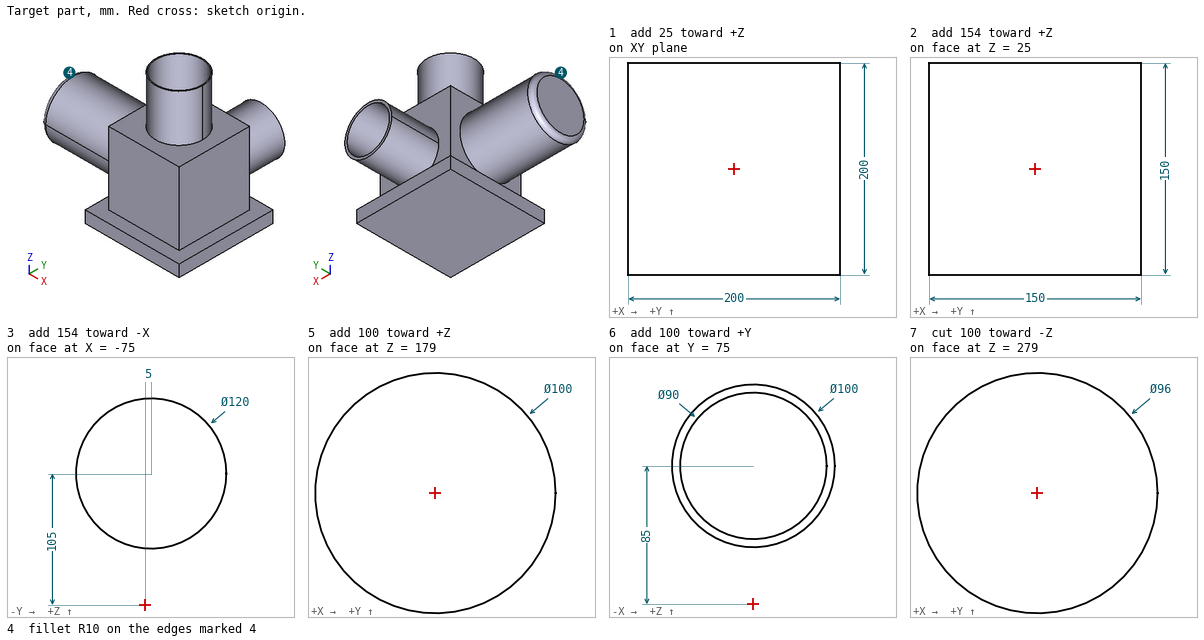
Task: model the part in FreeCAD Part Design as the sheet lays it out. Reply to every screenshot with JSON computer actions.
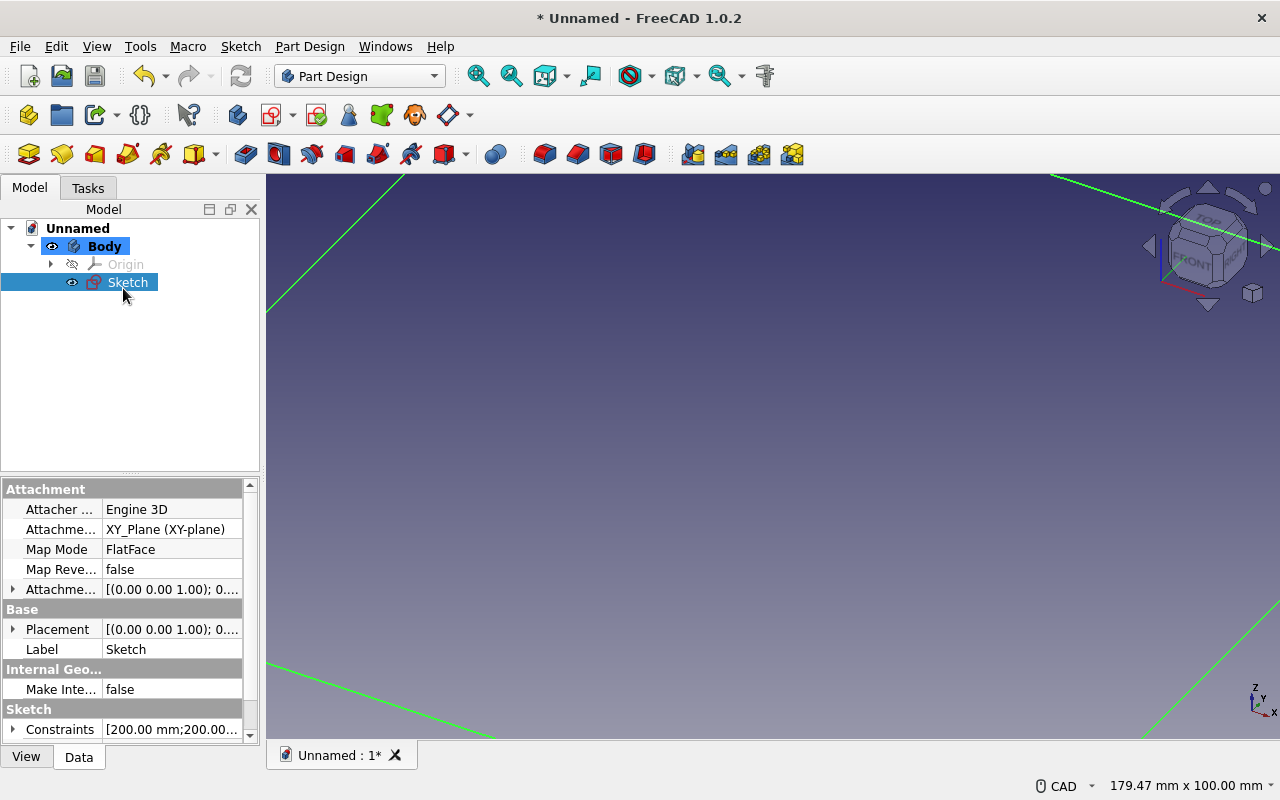
{"action": "left_click", "coordinate": [29, 154]}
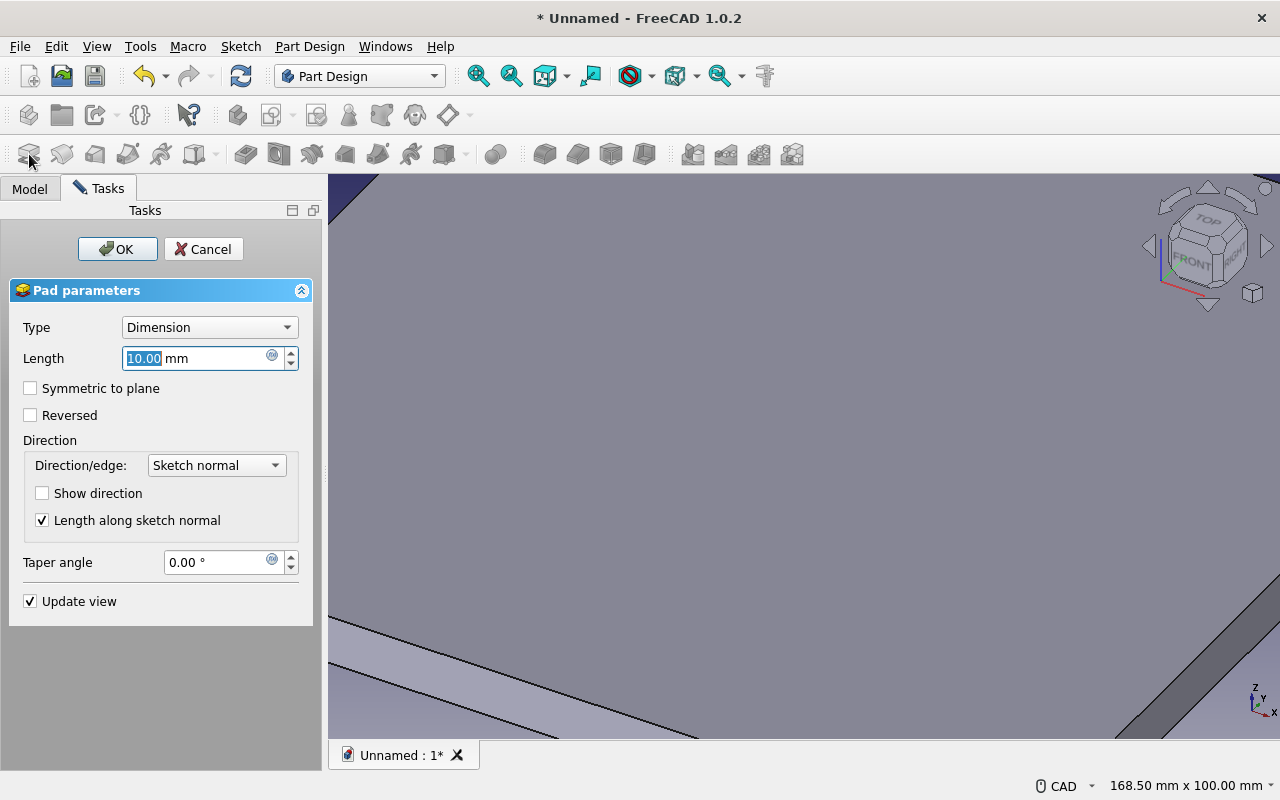
{"action": "type", "text": "25"}
{"action": "key", "text": "Tab"}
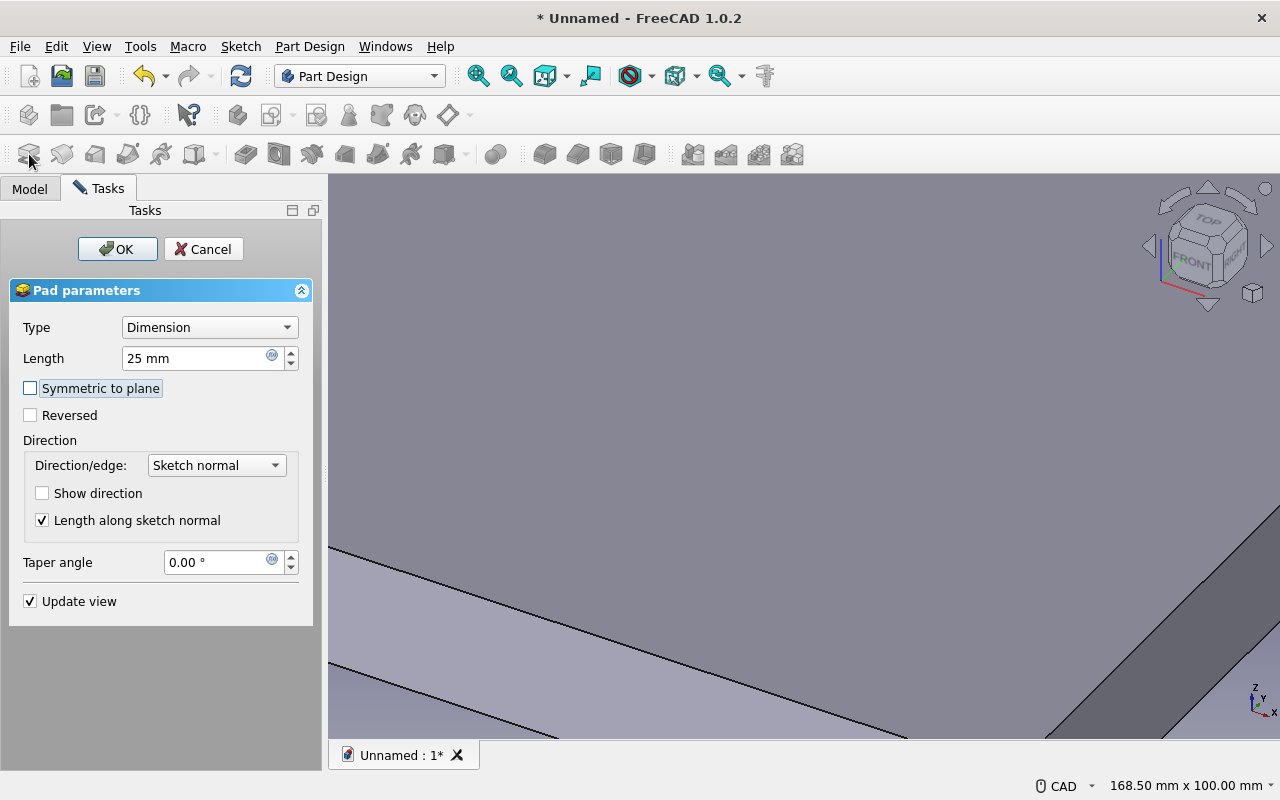
{"action": "left_click", "coordinate": [118, 249]}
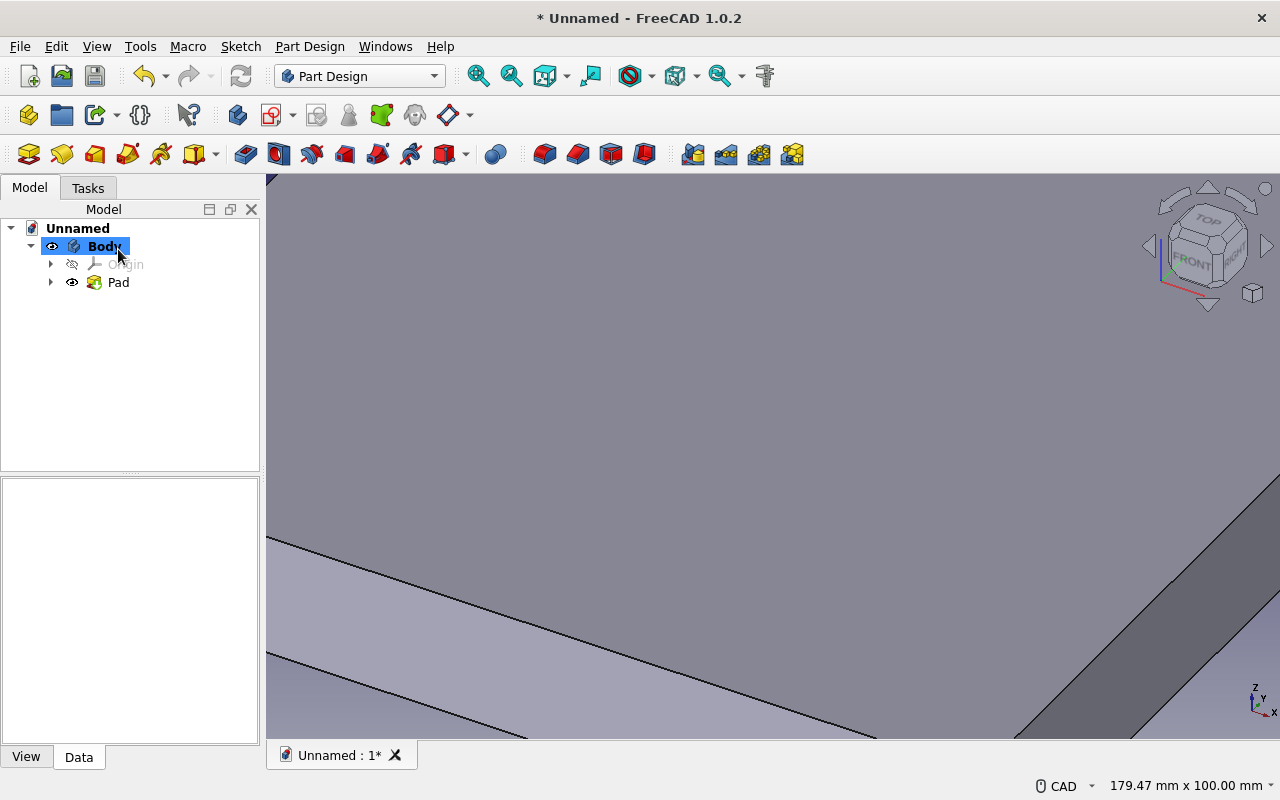
{"action": "left_click", "coordinate": [479, 76]}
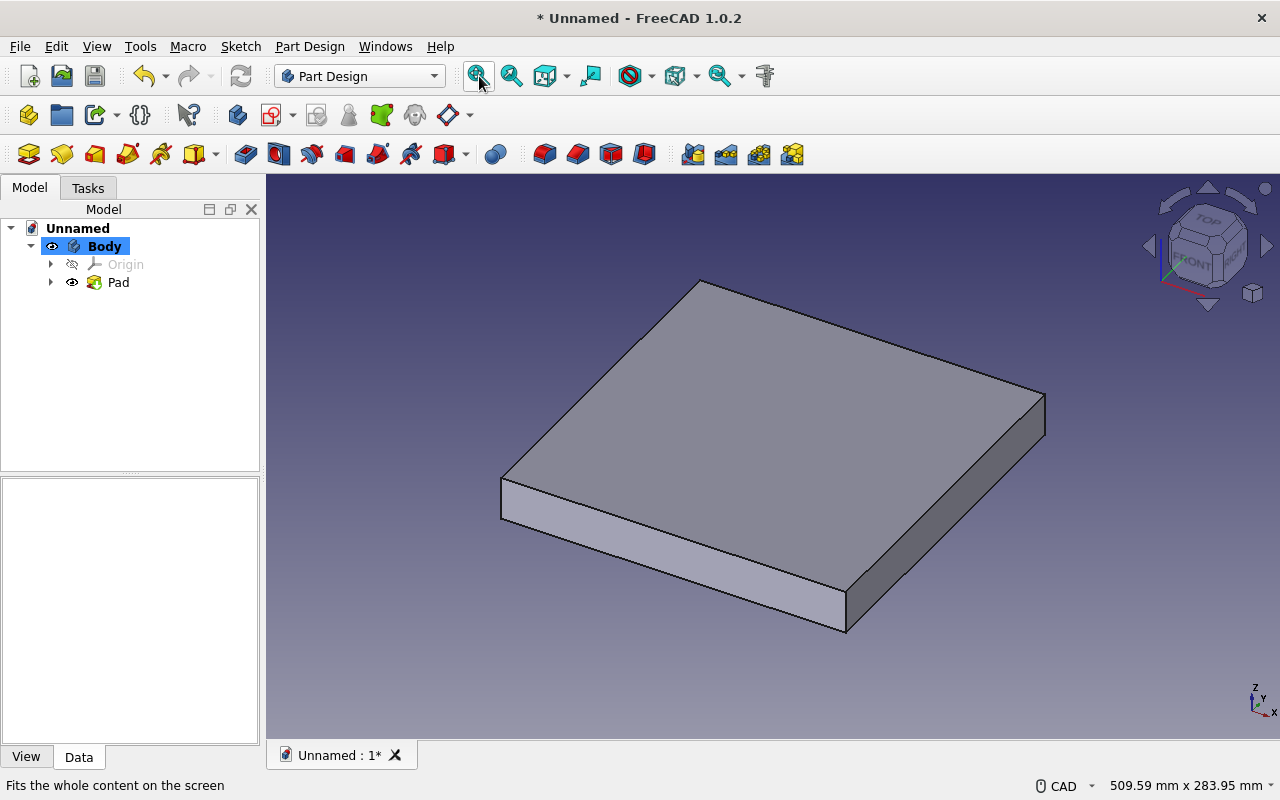
{"action": "left_click", "coordinate": [773, 435]}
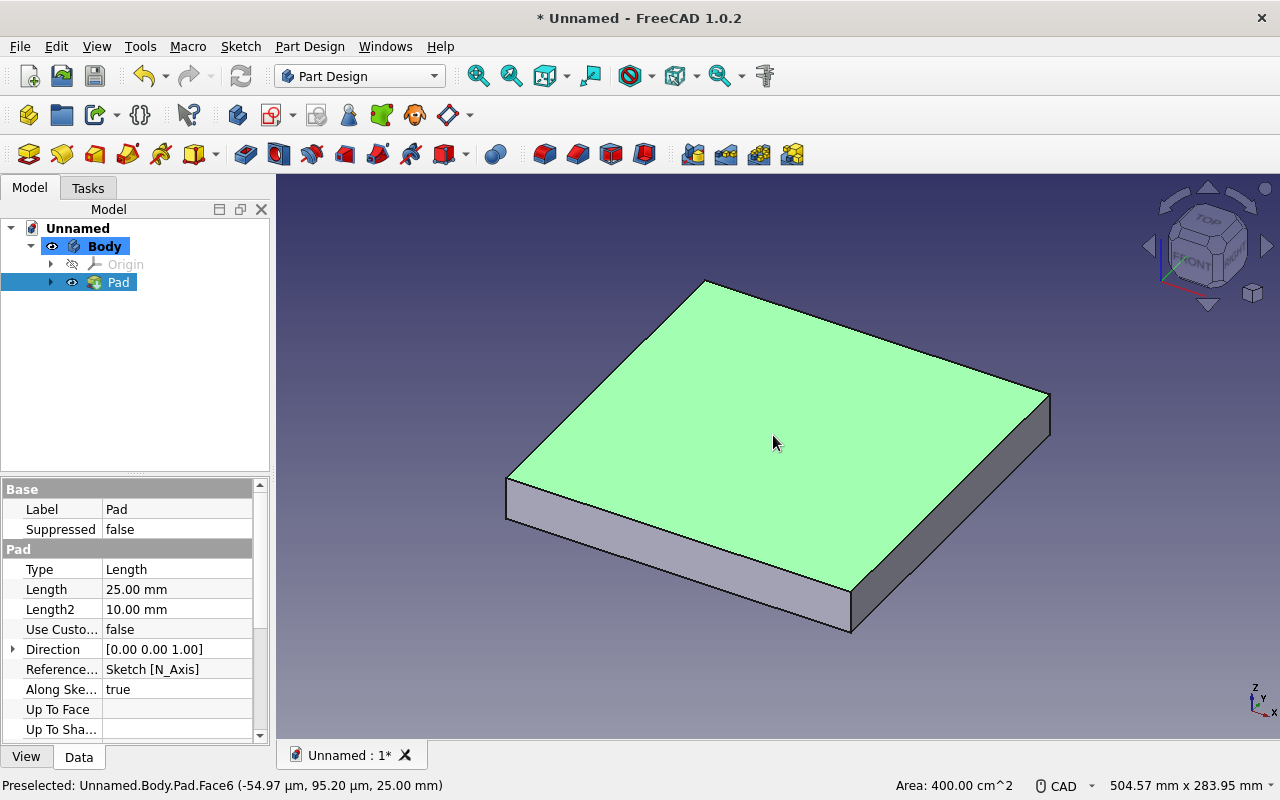
{"action": "left_click", "coordinate": [270, 116]}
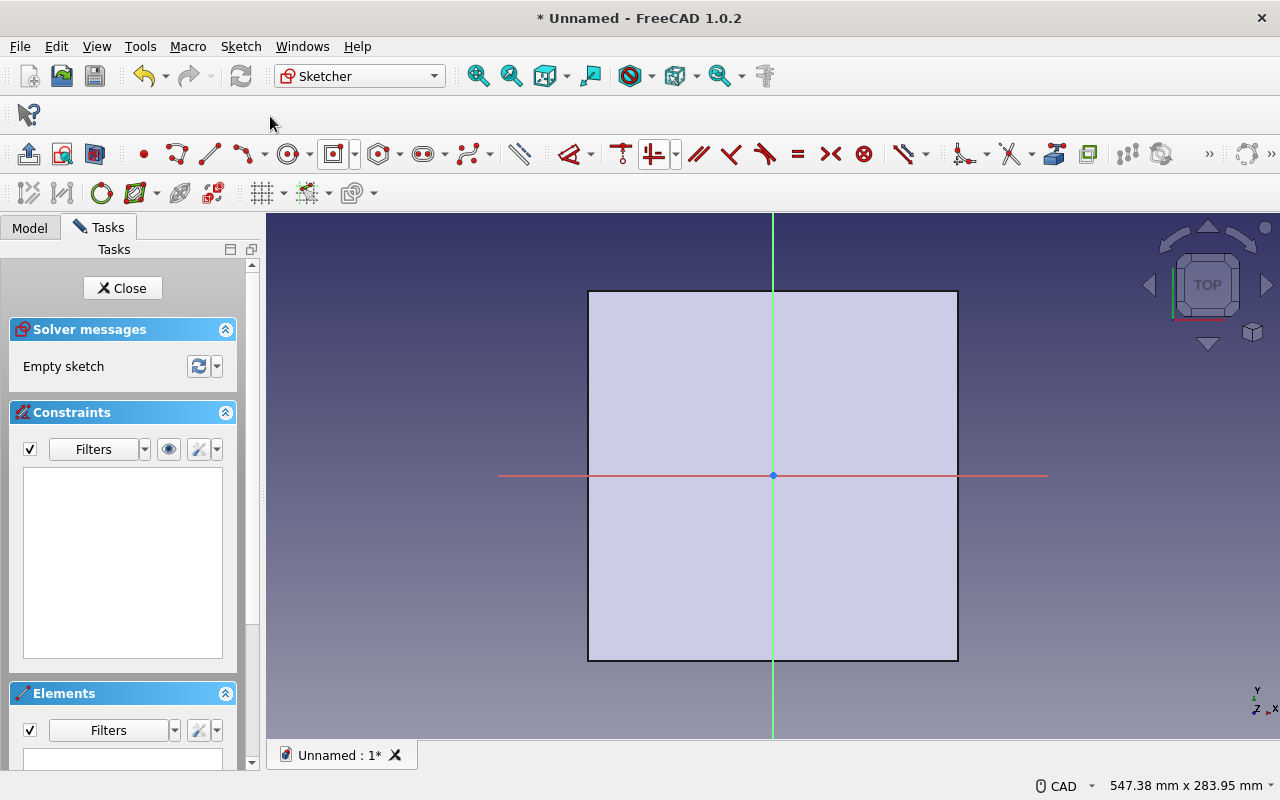
{"action": "left_click", "coordinate": [332, 154]}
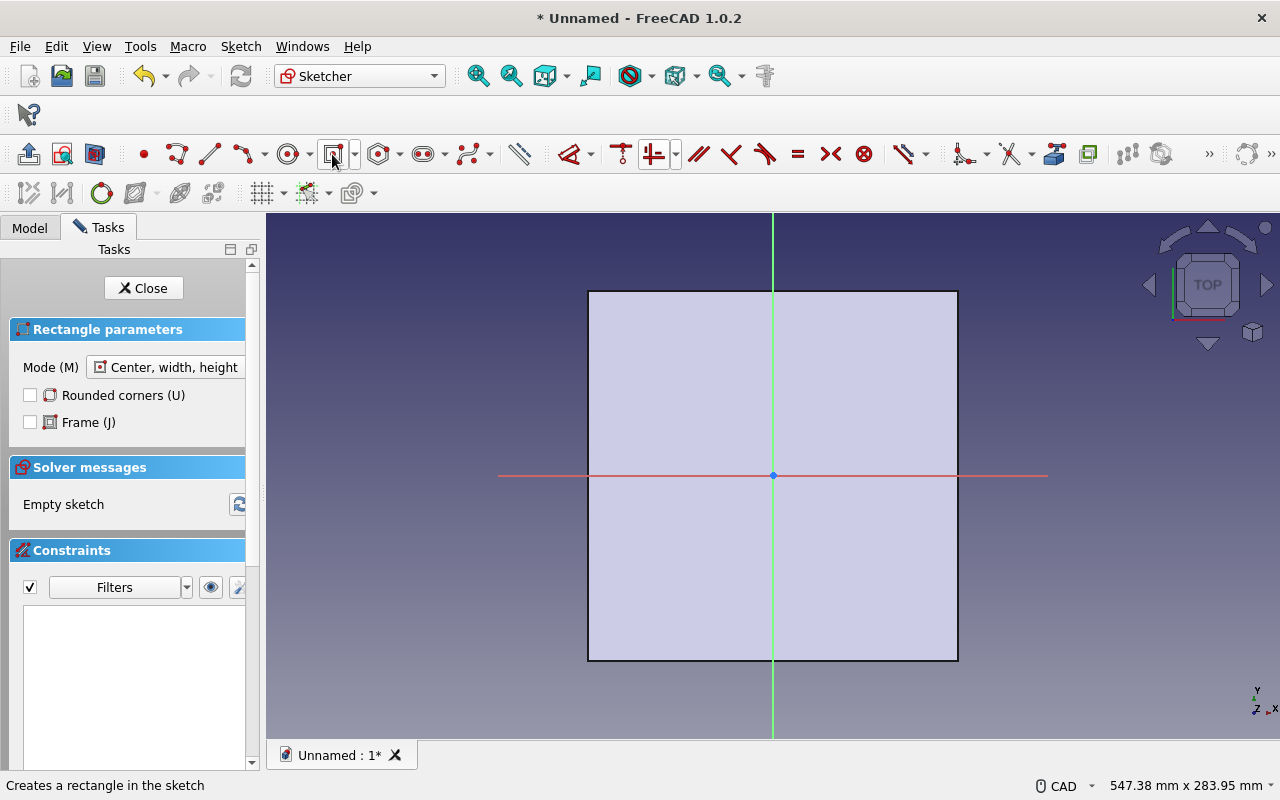
{"action": "left_click", "coordinate": [773, 476]}
{"action": "mouse_move", "coordinate": [912, 337]}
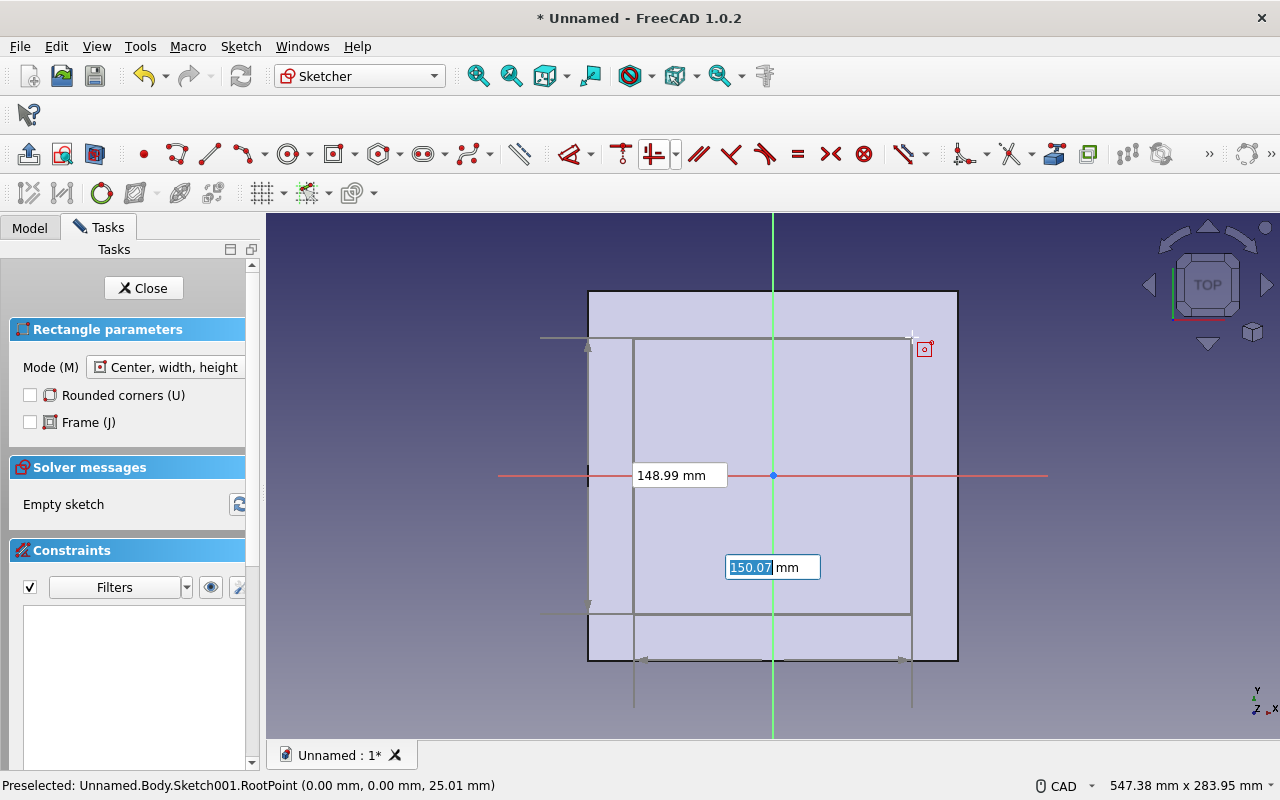
{"action": "type", "text": "150"}
{"action": "key", "text": "Tab"}
{"action": "type", "text": "150"}
{"action": "key", "text": "Return"}
{"action": "key", "text": "Escape"}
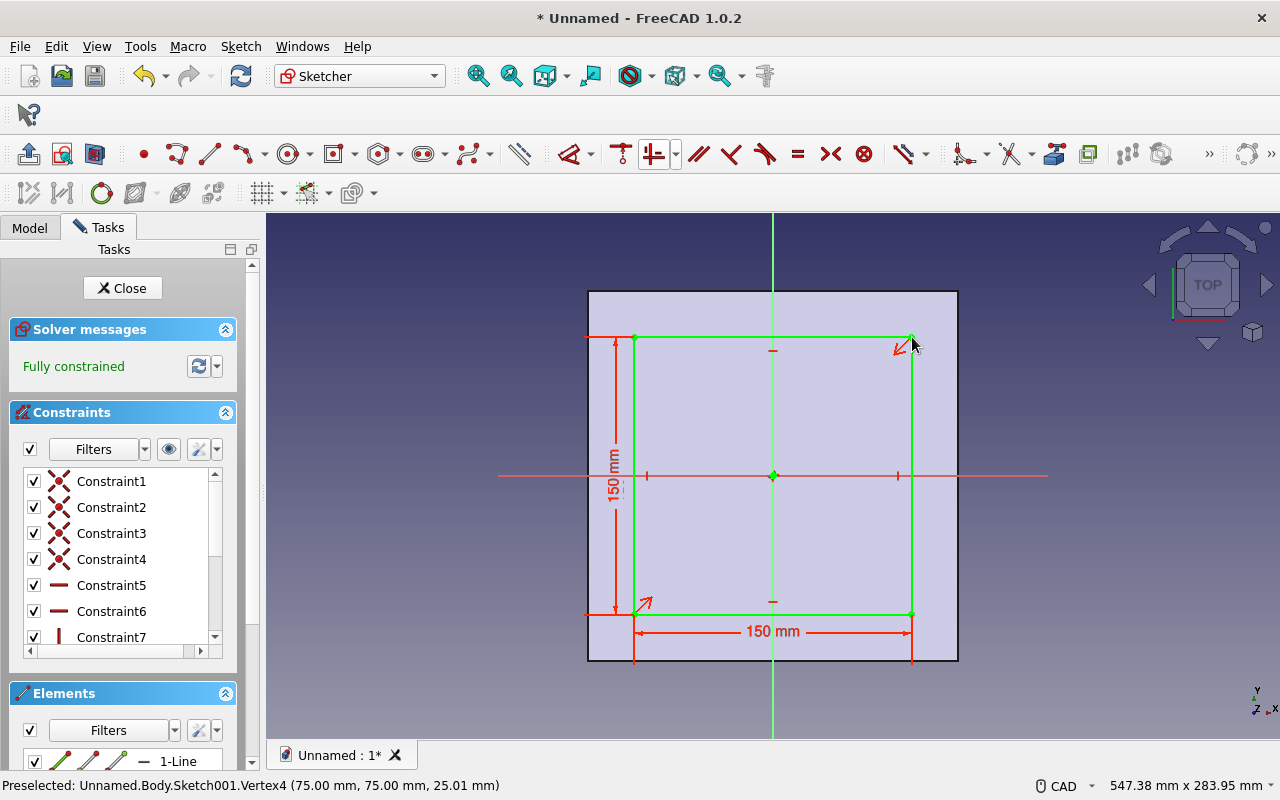
{"action": "left_click", "coordinate": [123, 288]}